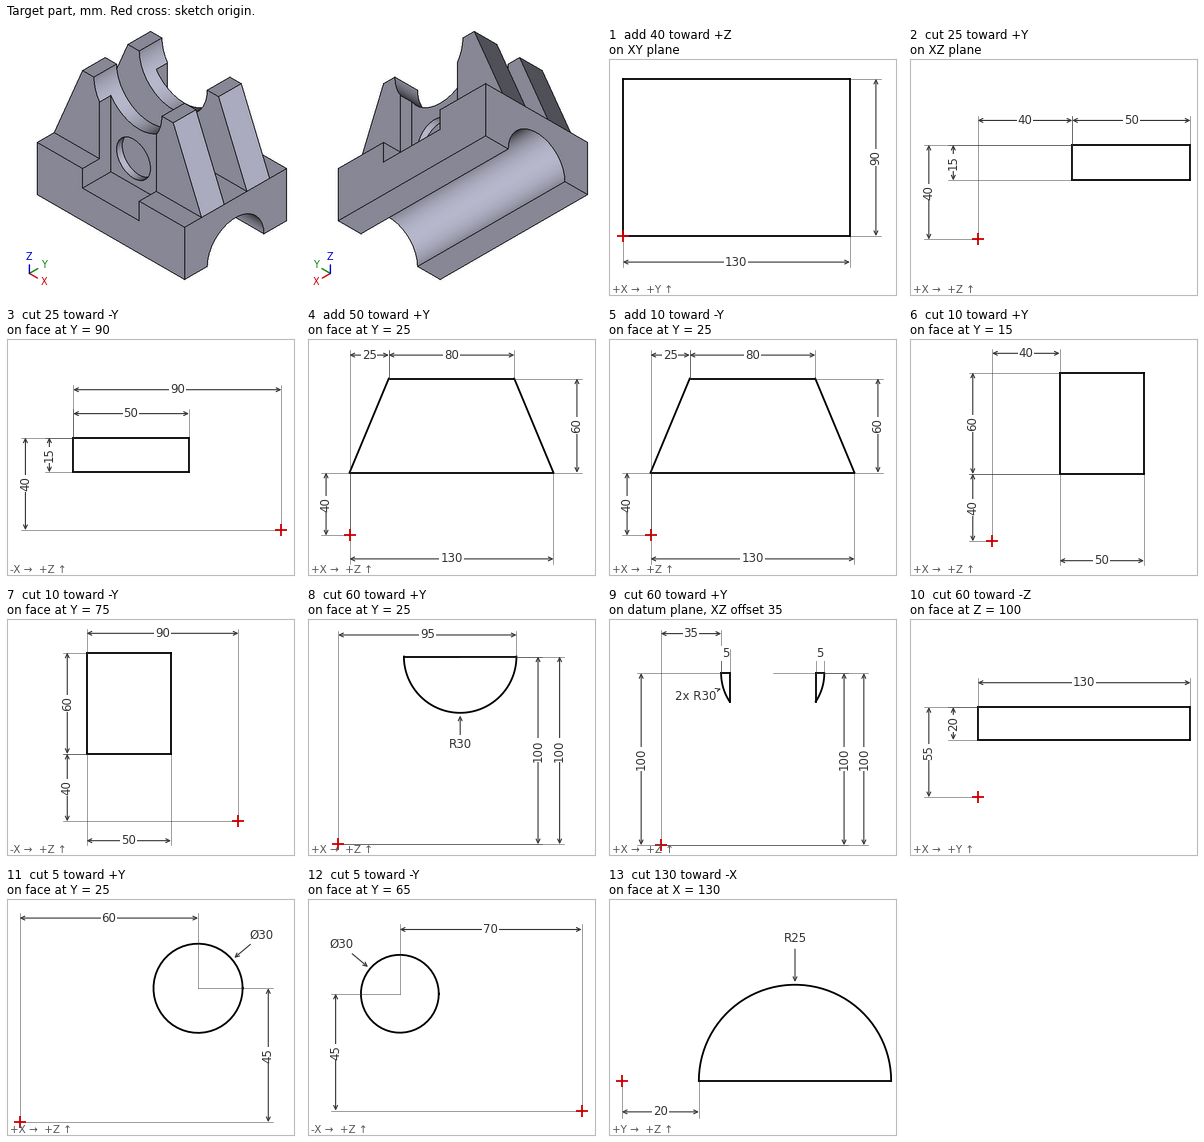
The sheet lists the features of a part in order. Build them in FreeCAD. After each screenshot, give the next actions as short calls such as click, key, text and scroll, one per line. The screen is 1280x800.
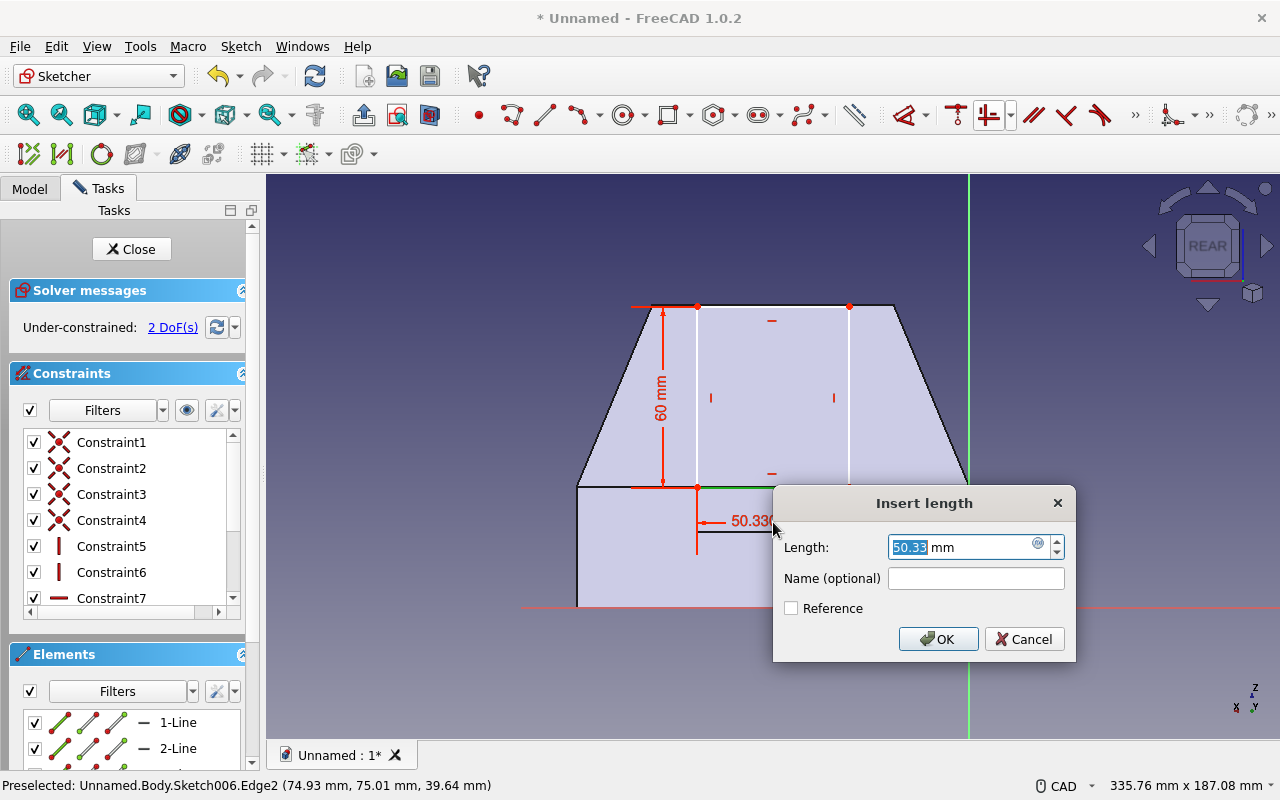
text(50)
key(Return)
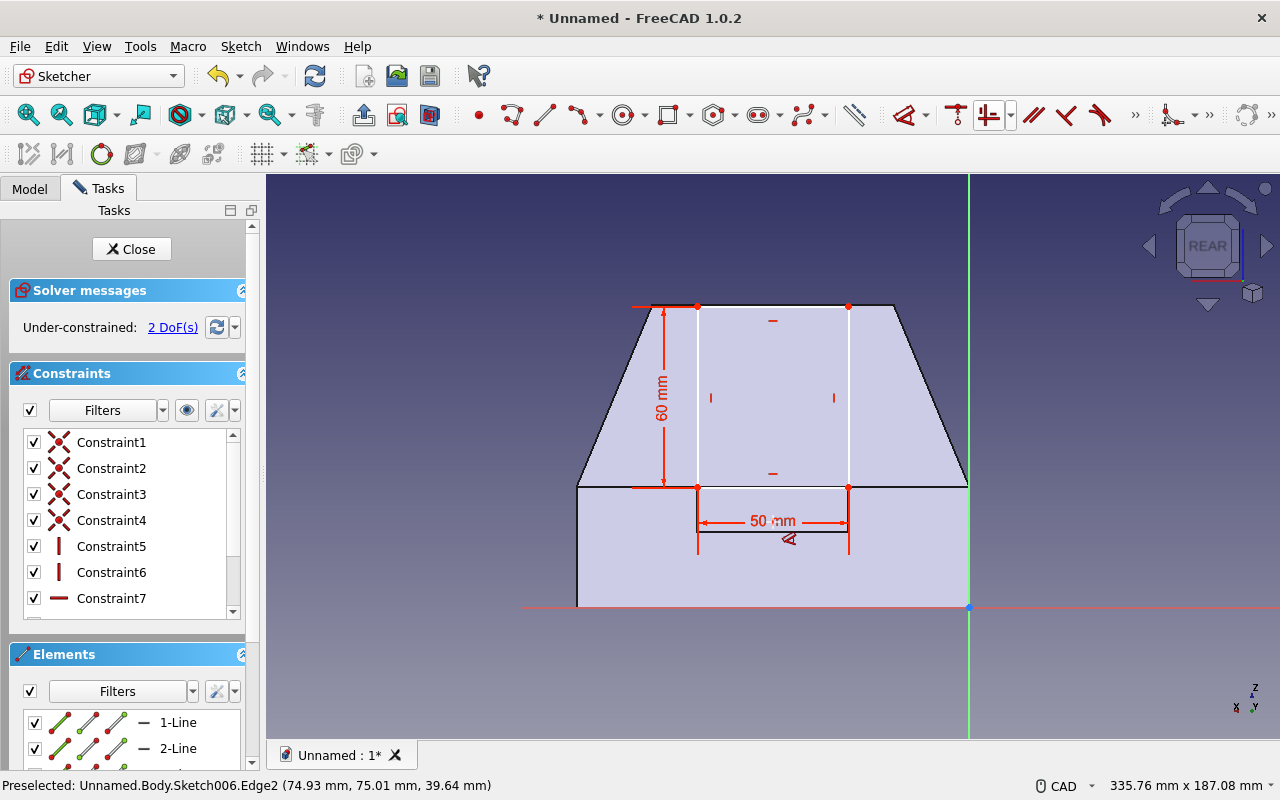
click(698, 307)
click(834, 642)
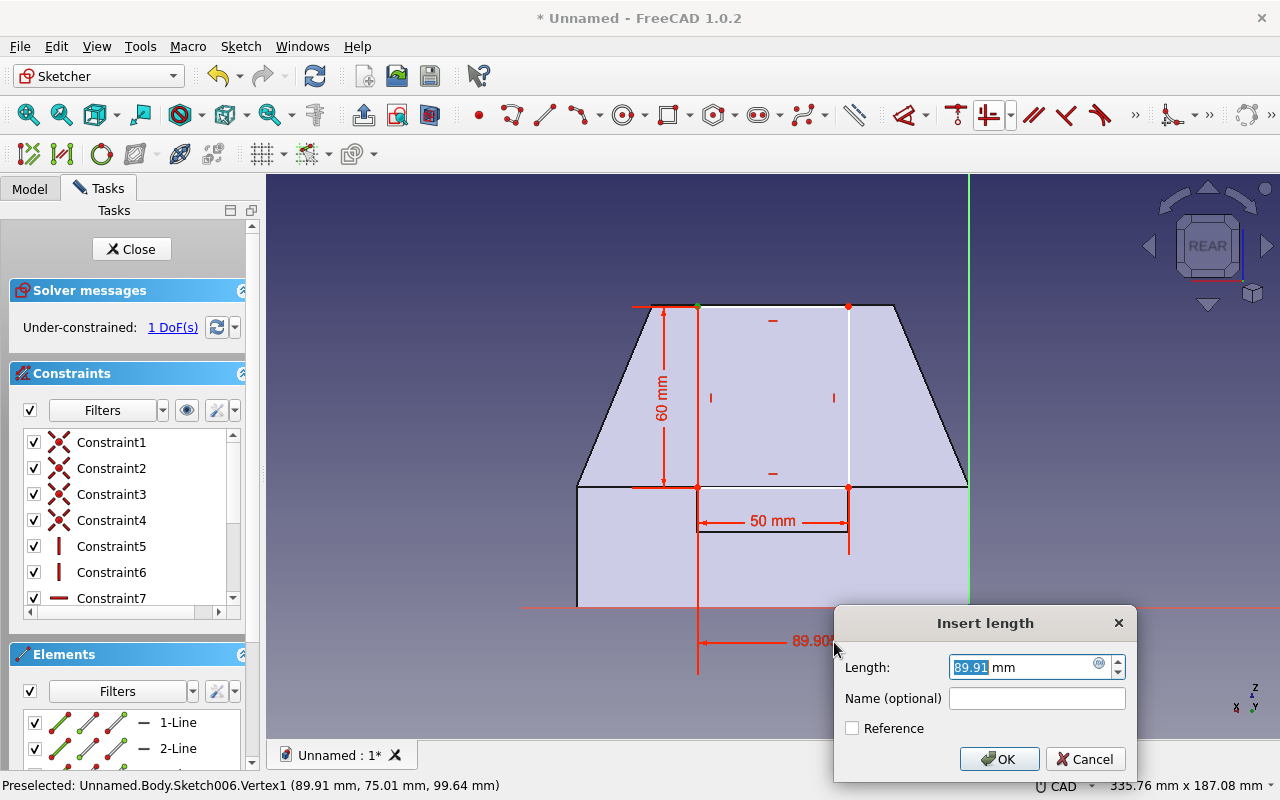
text(90)
key(Return)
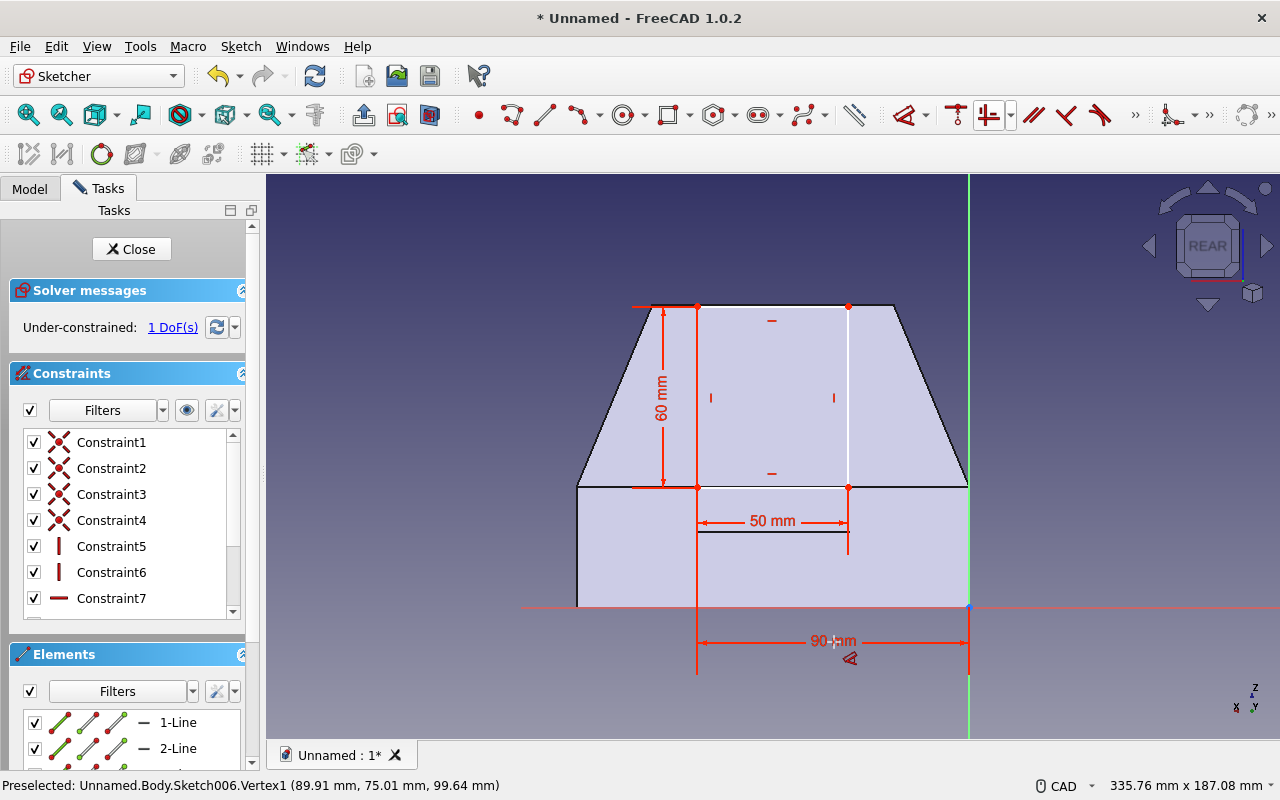
click(697, 488)
click(1003, 548)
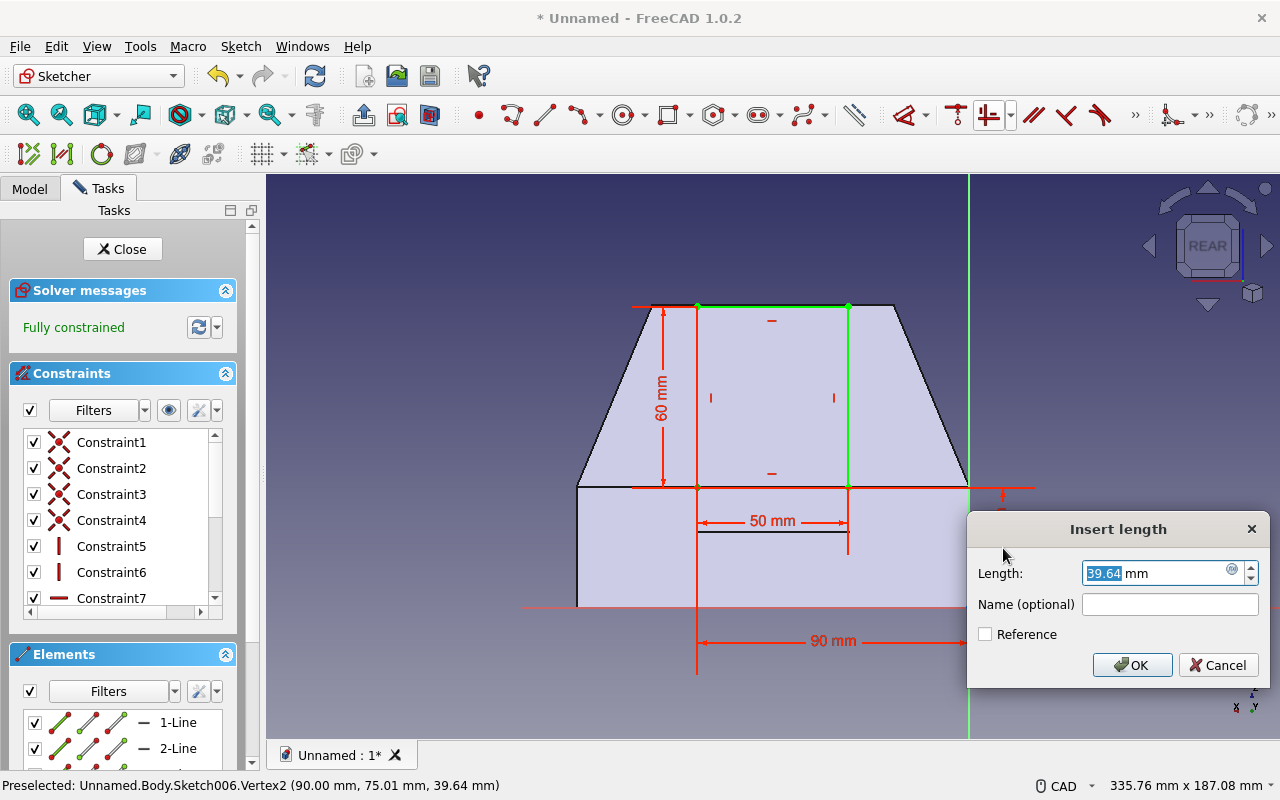
text(40)
key(Return)
key(Escape)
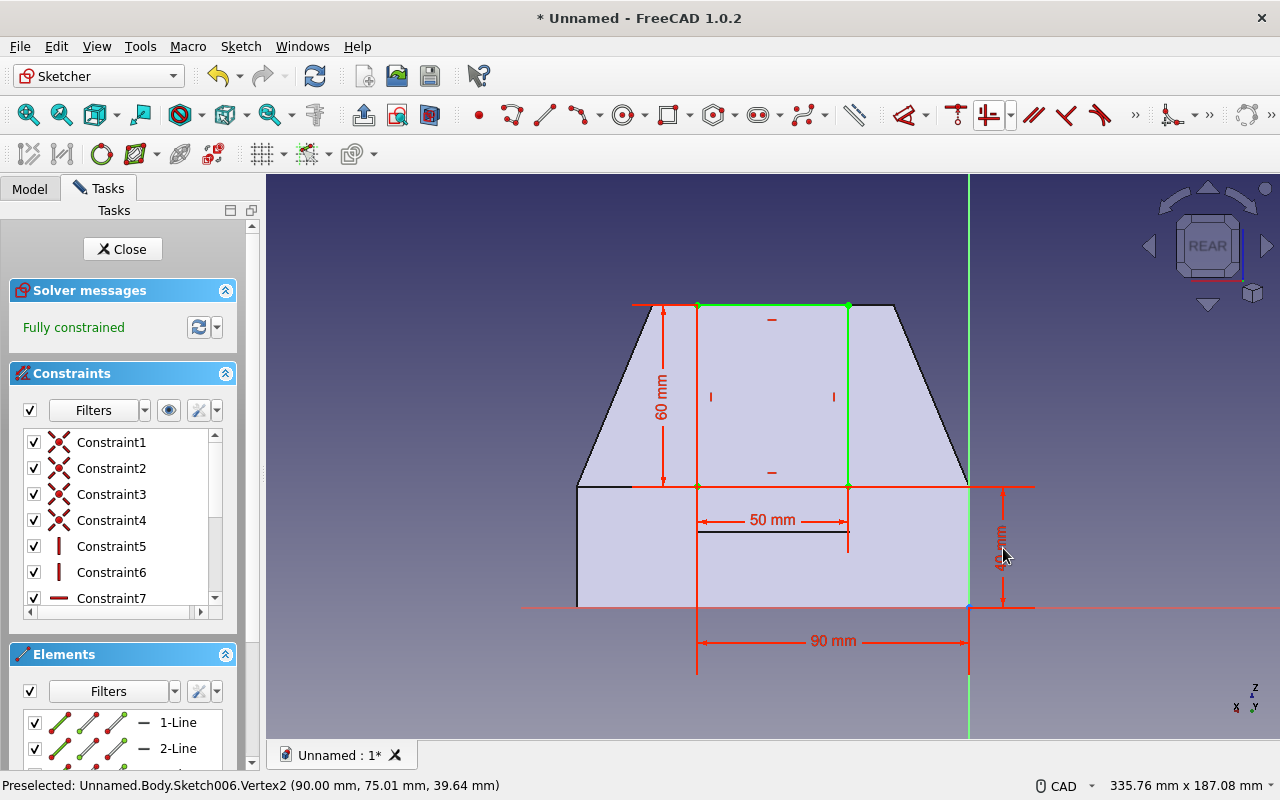
click(123, 249)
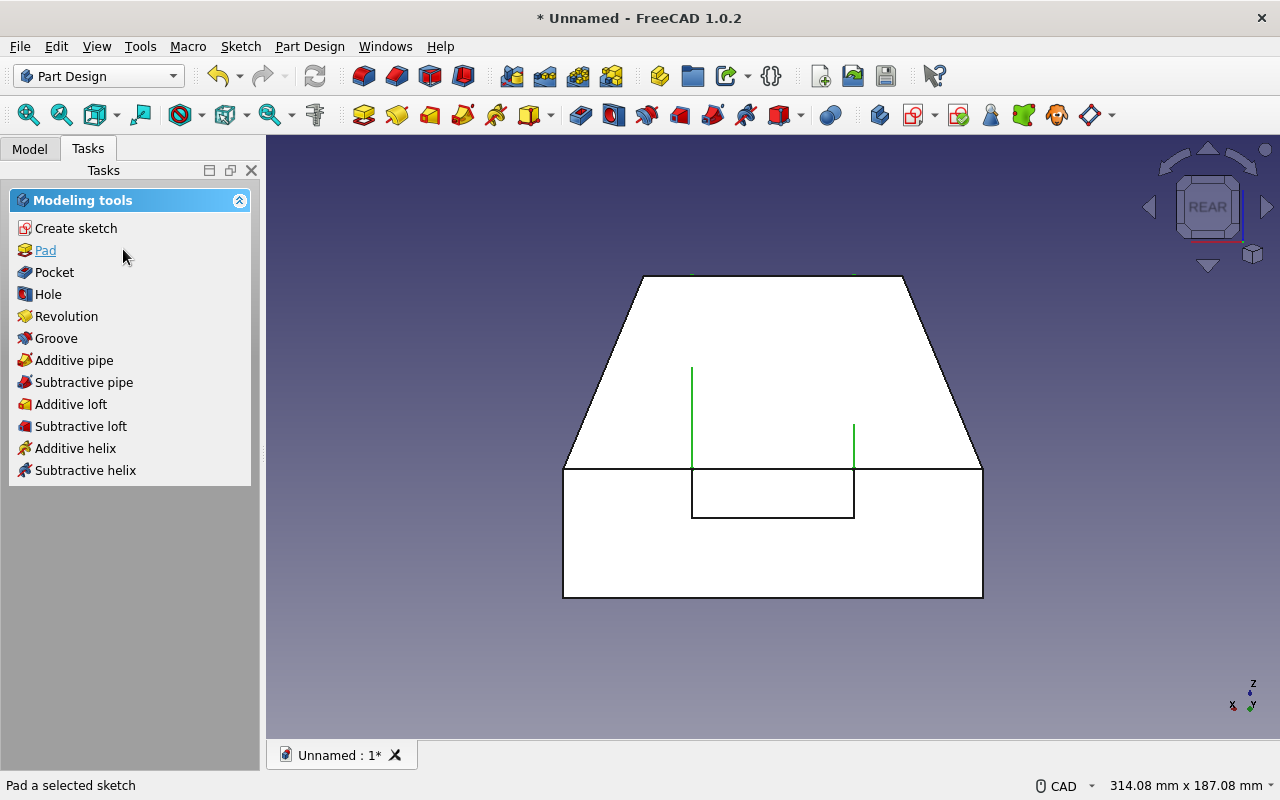
click(581, 116)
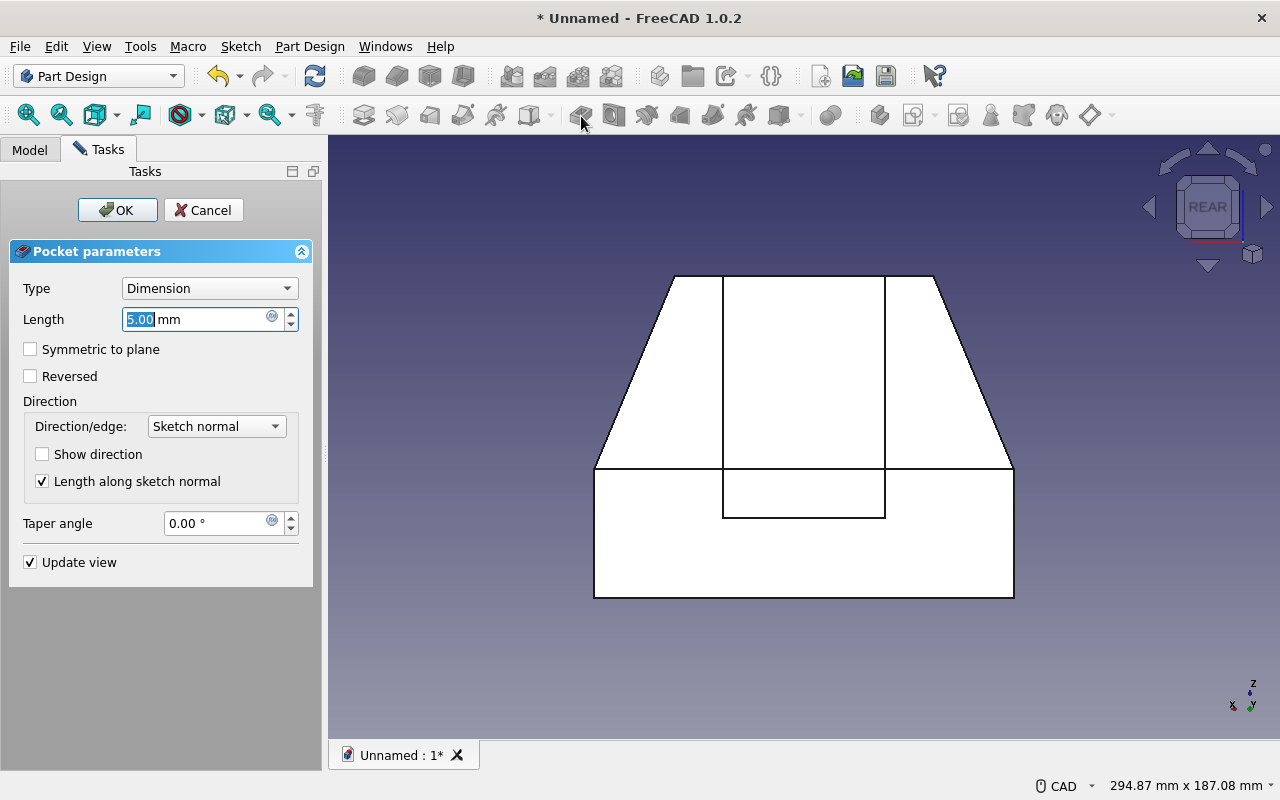
text(10)
key(Tab)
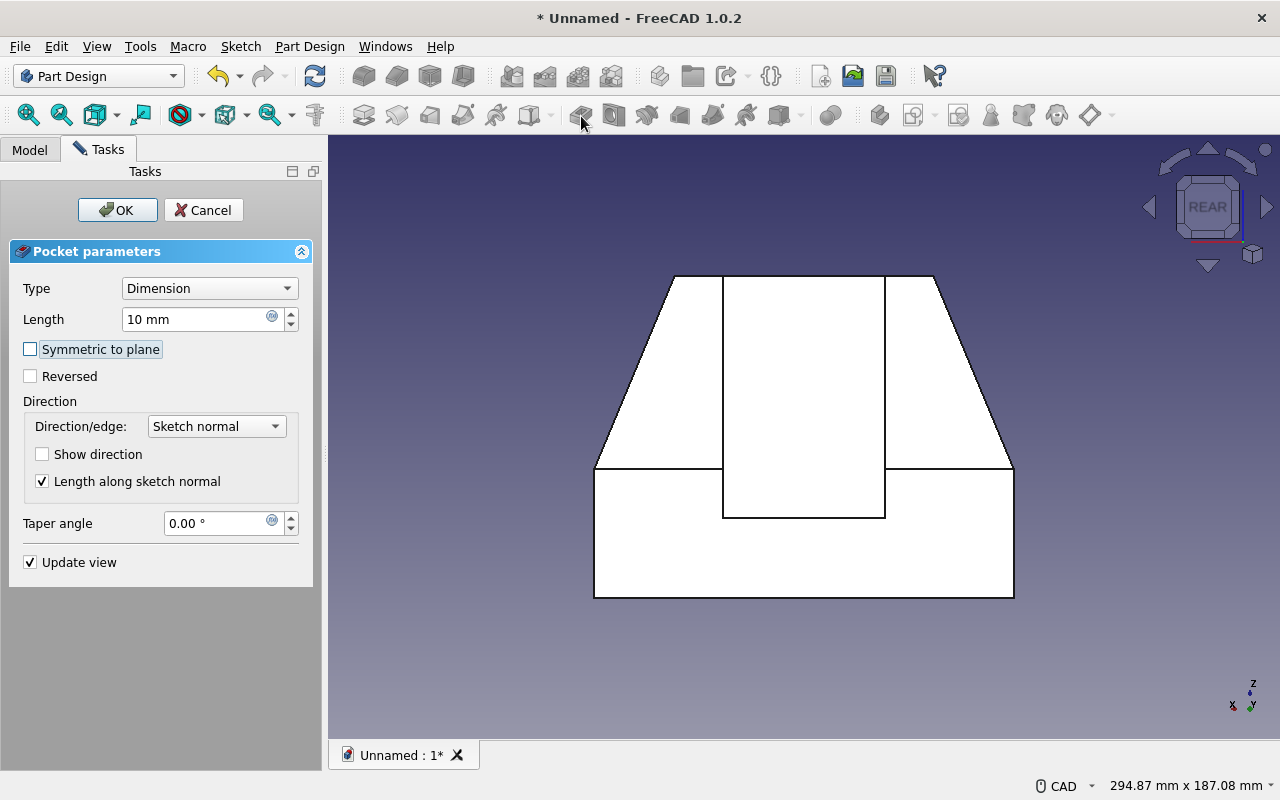
click(118, 210)